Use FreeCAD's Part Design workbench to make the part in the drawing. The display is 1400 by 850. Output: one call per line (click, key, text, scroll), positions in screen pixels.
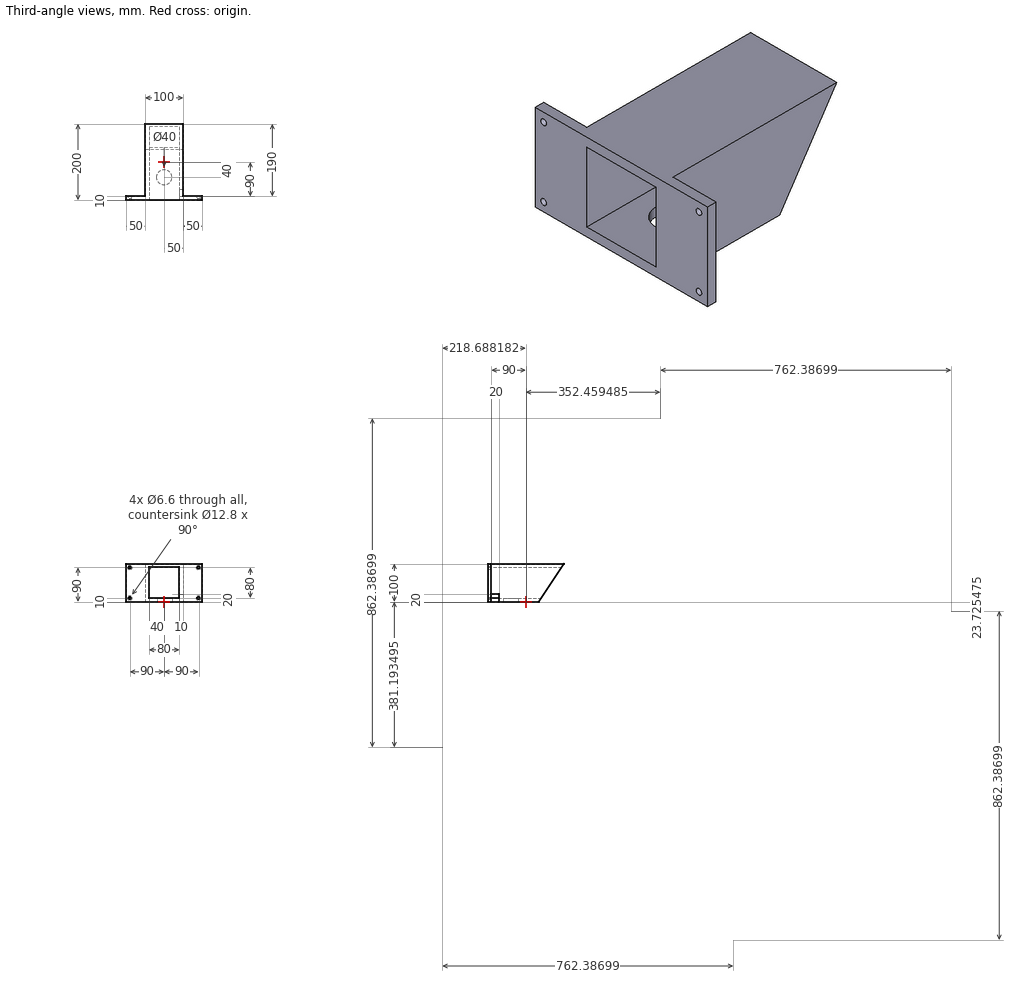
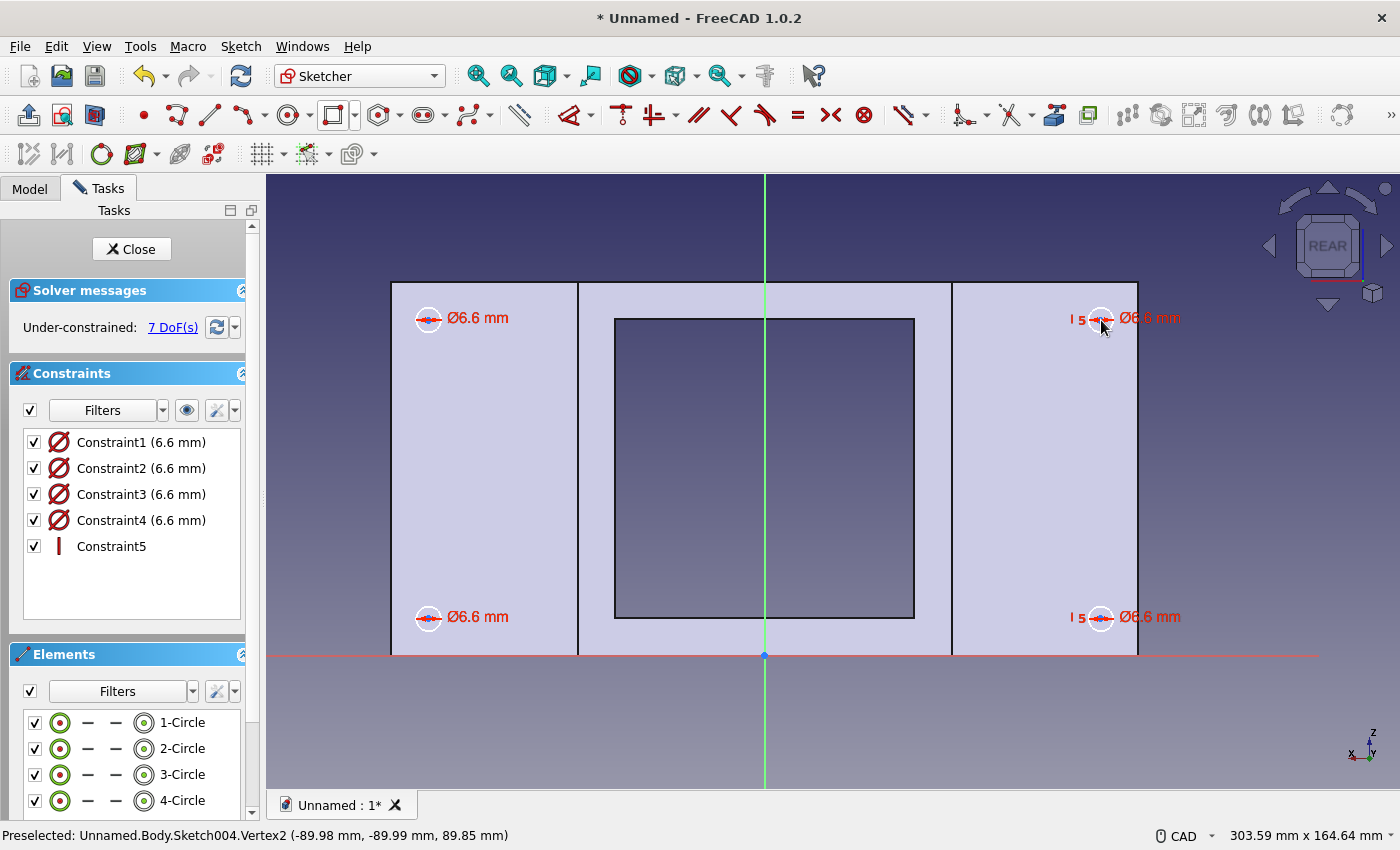
click(1101, 619)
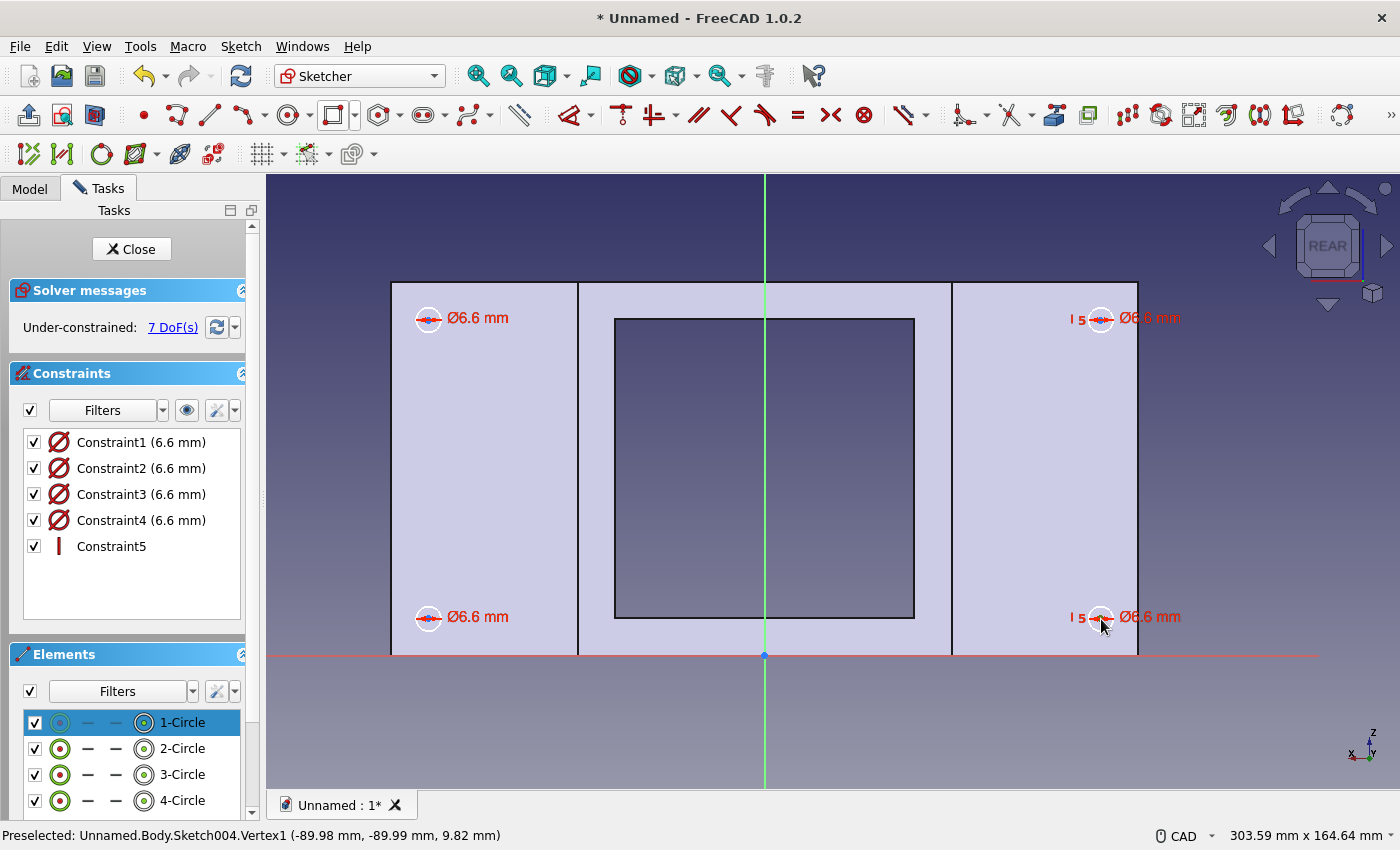
click(429, 619)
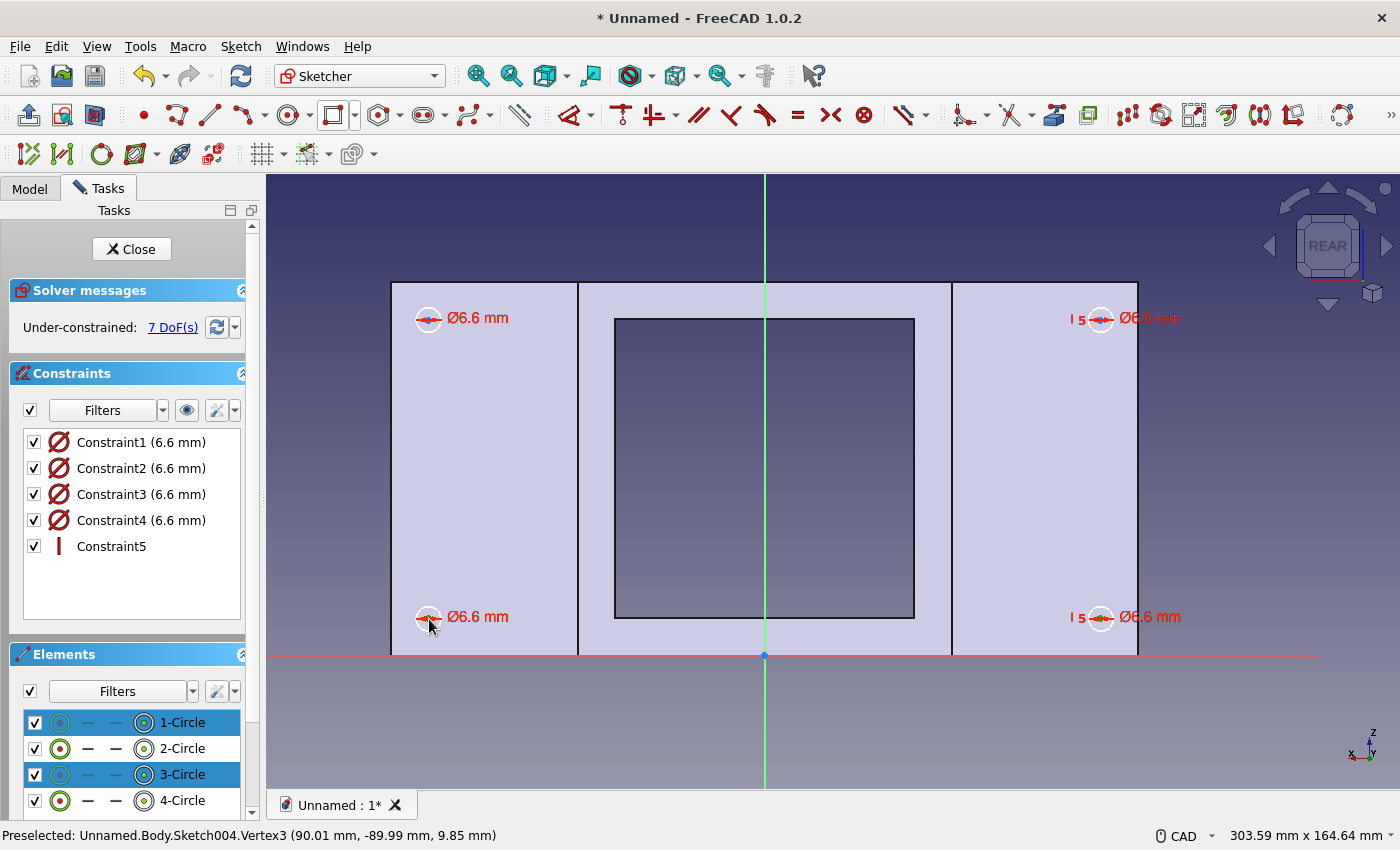
key(h)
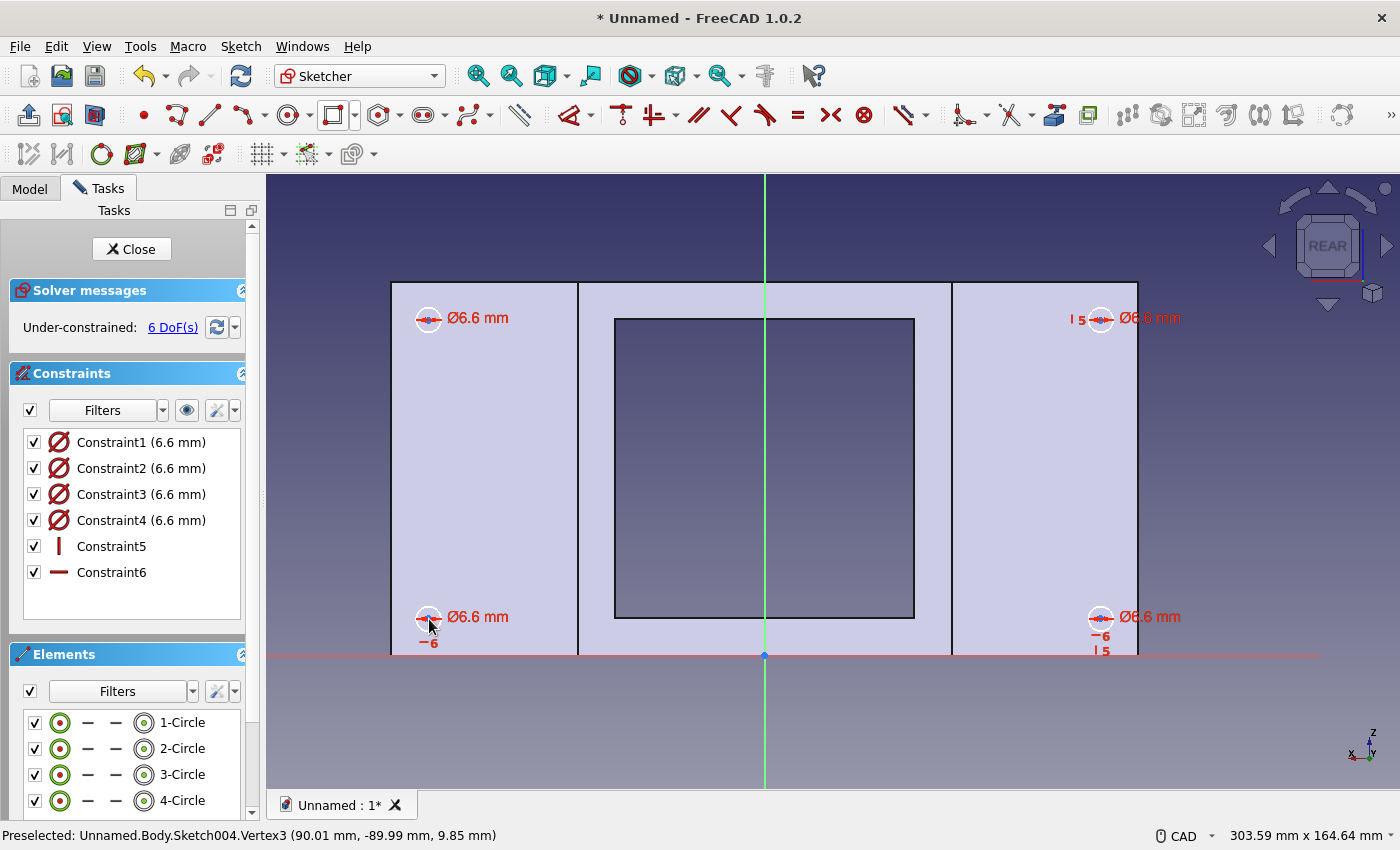
click(429, 619)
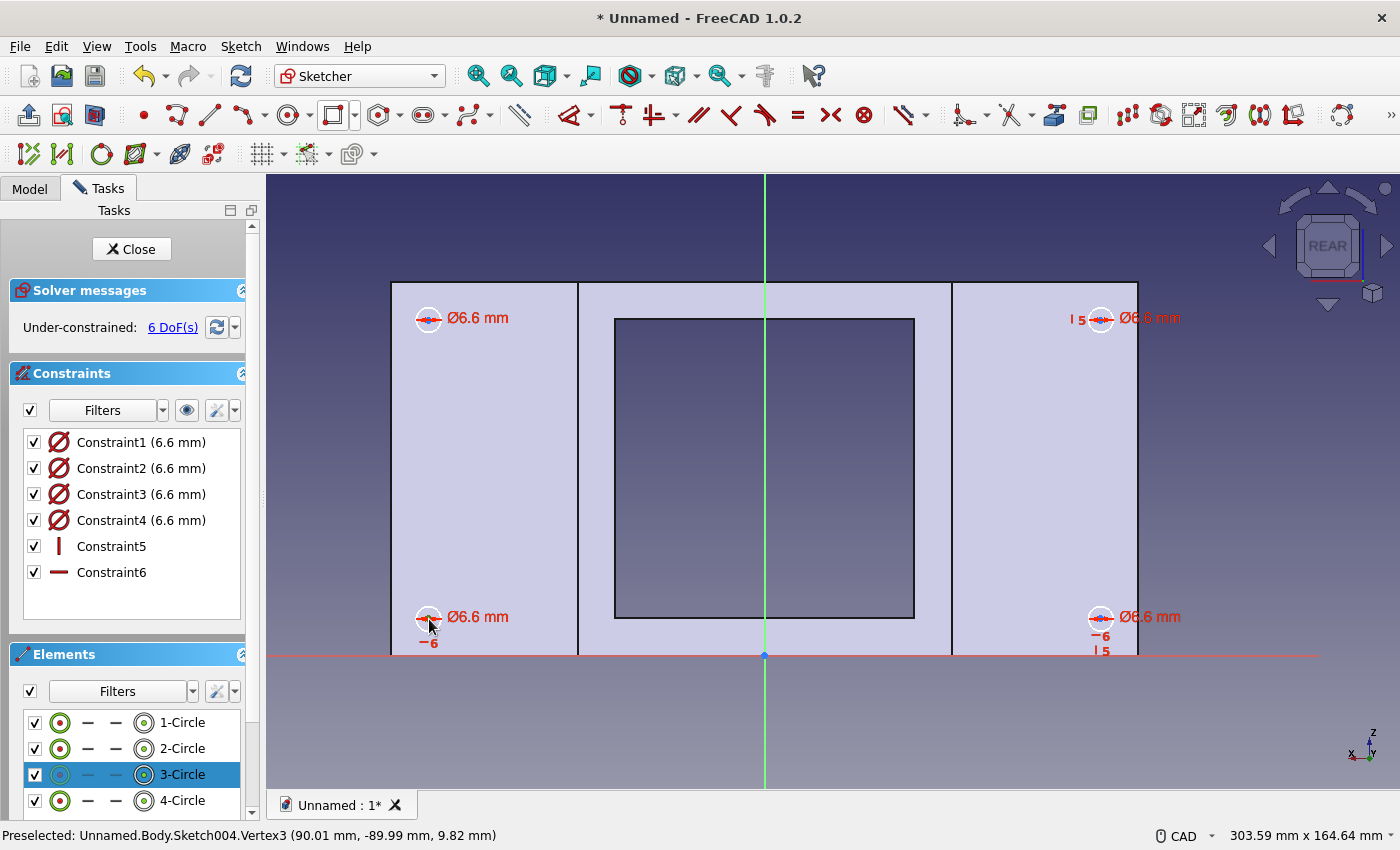
click(429, 320)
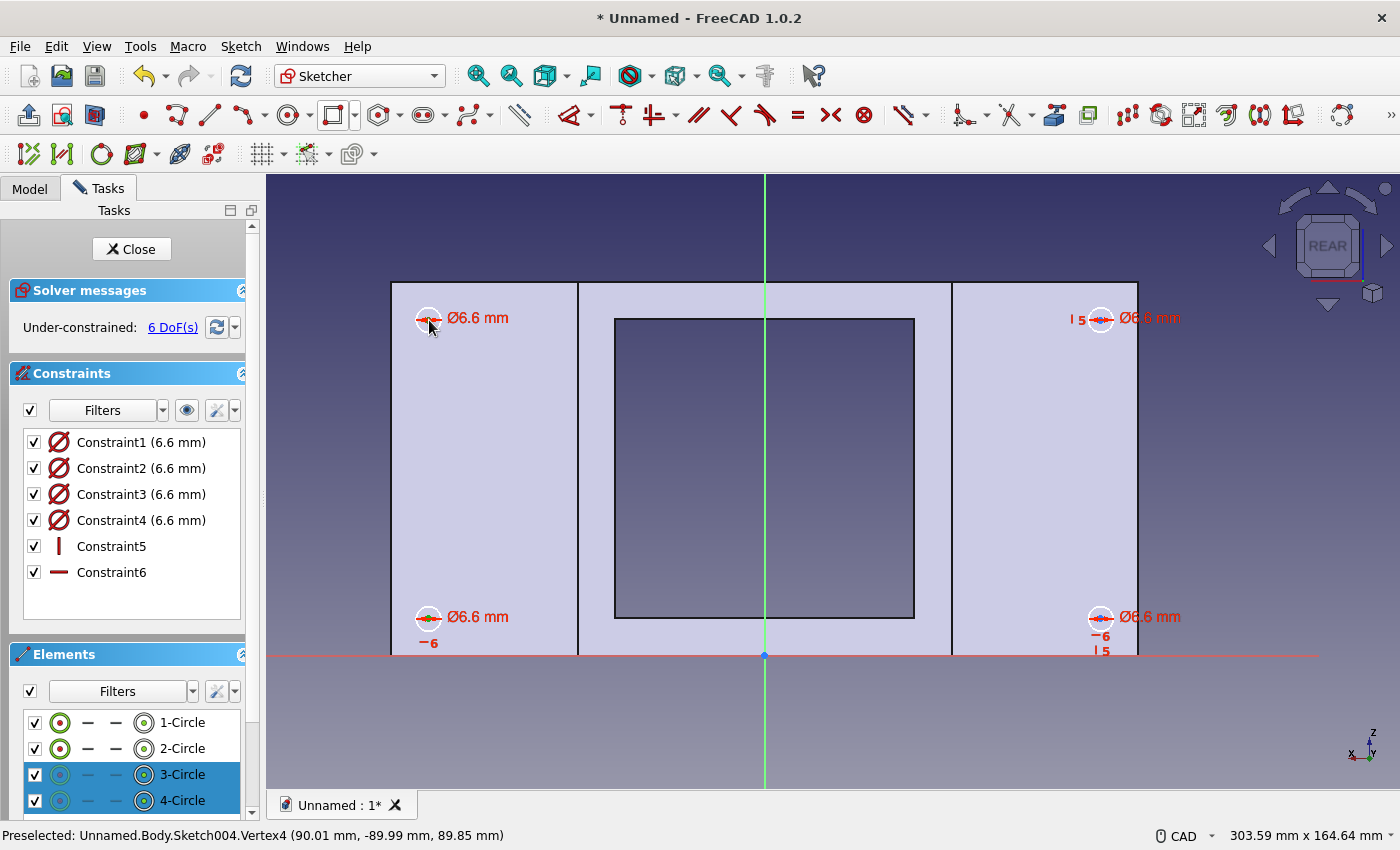
key(v)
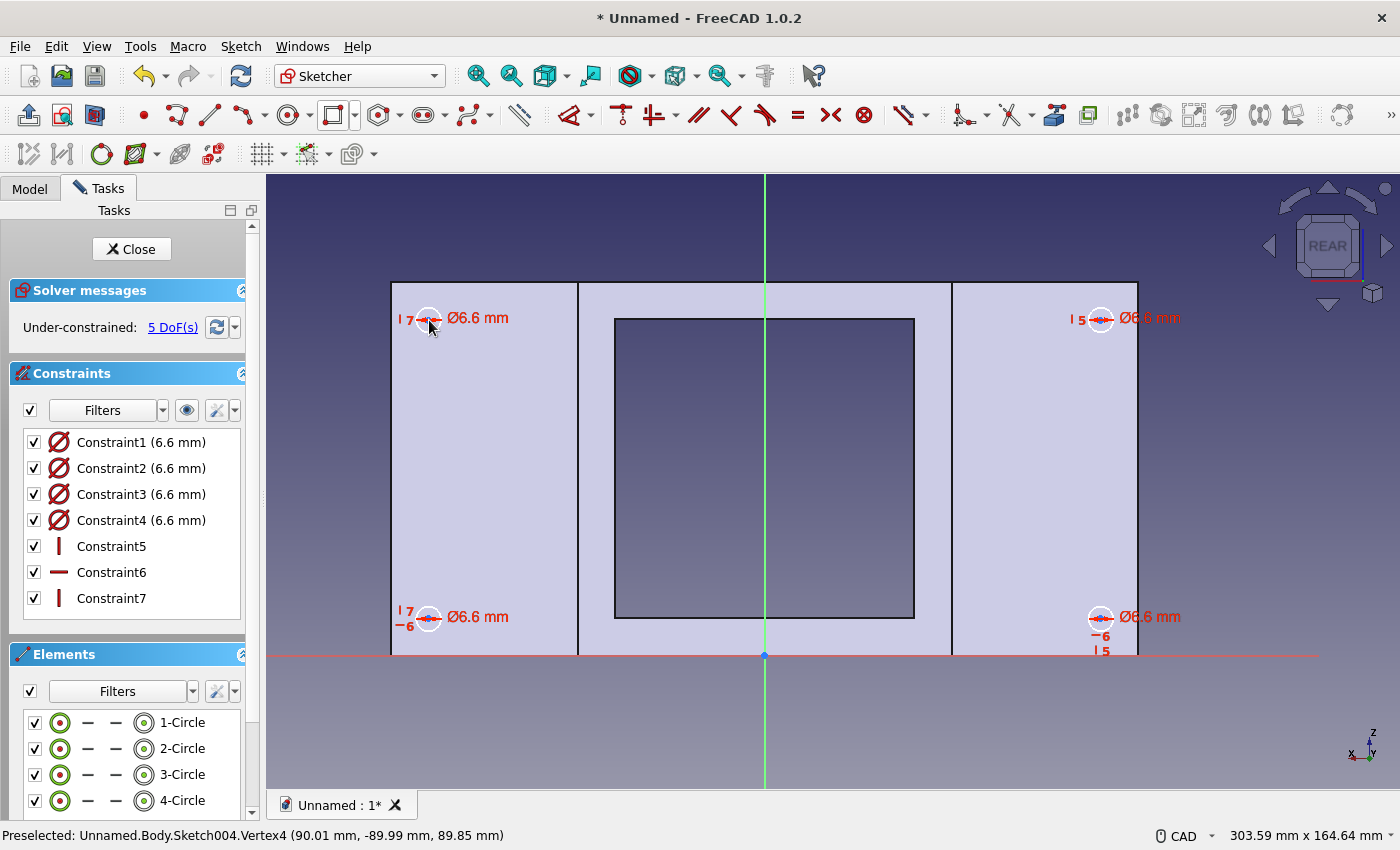
click(1101, 320)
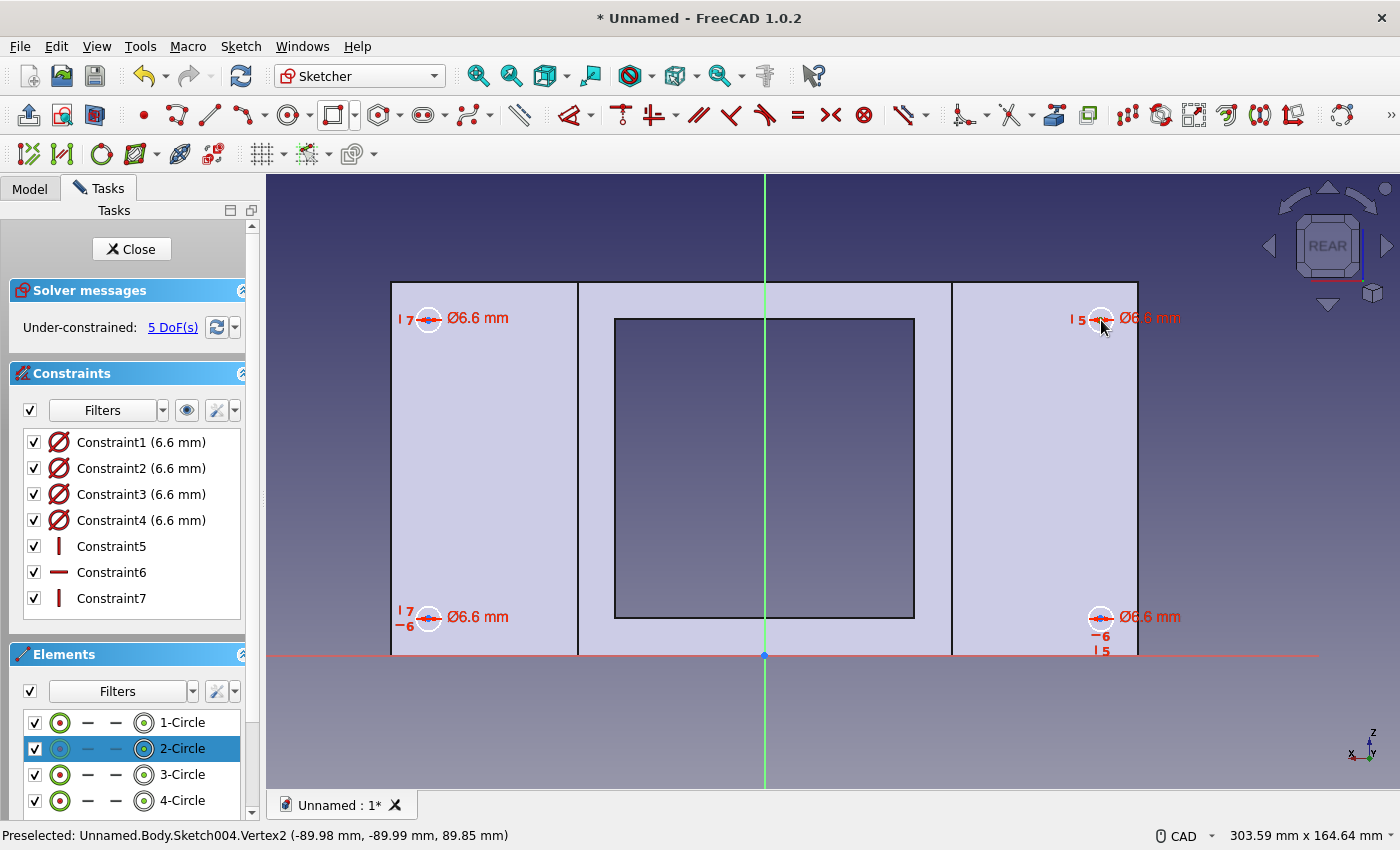
click(429, 320)